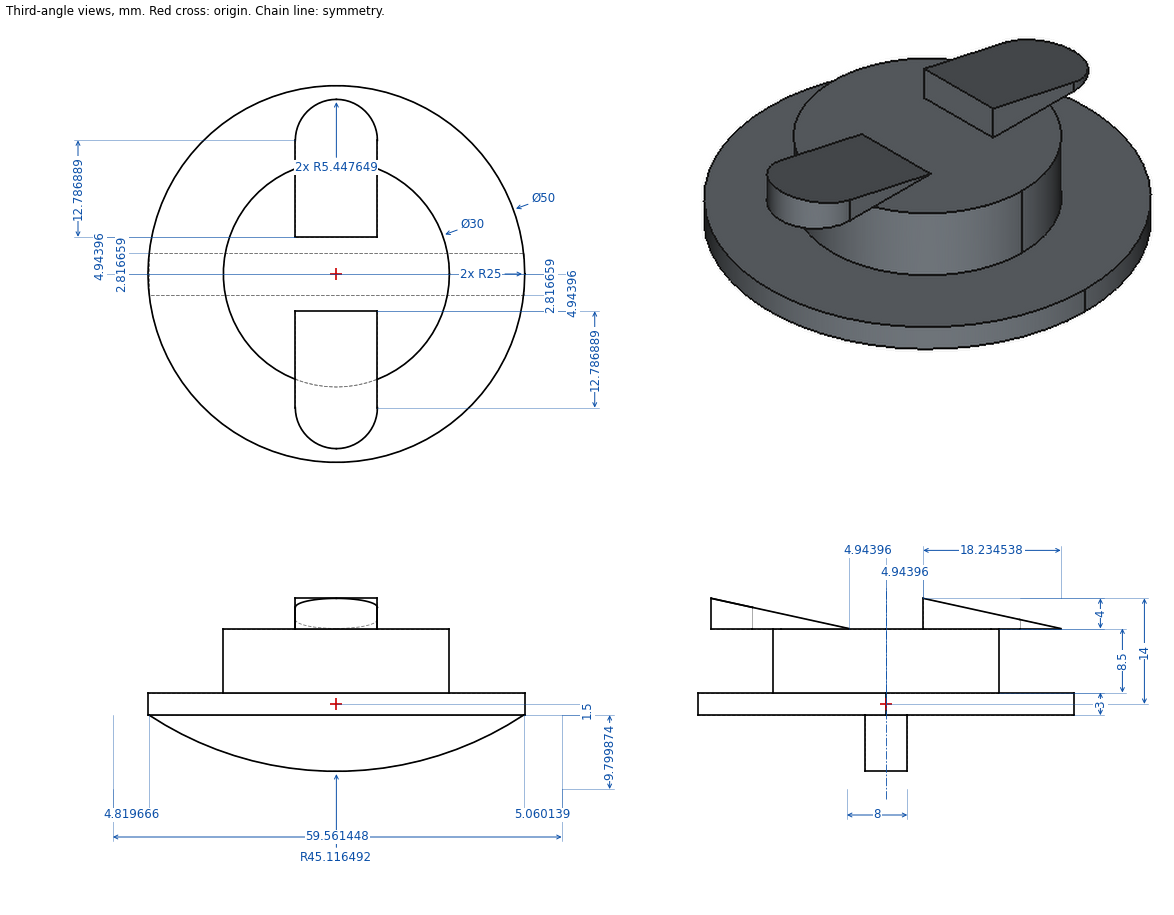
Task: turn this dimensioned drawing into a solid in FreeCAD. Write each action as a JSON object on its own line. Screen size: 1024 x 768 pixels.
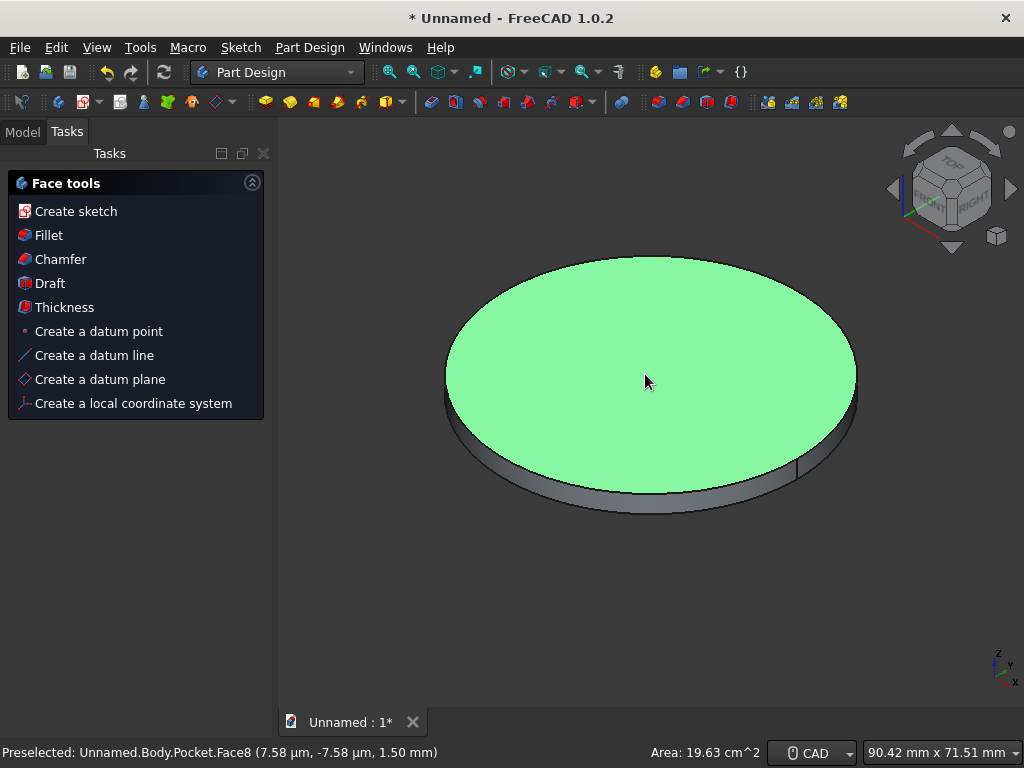
{"action": "left_click", "coordinate": [84, 102]}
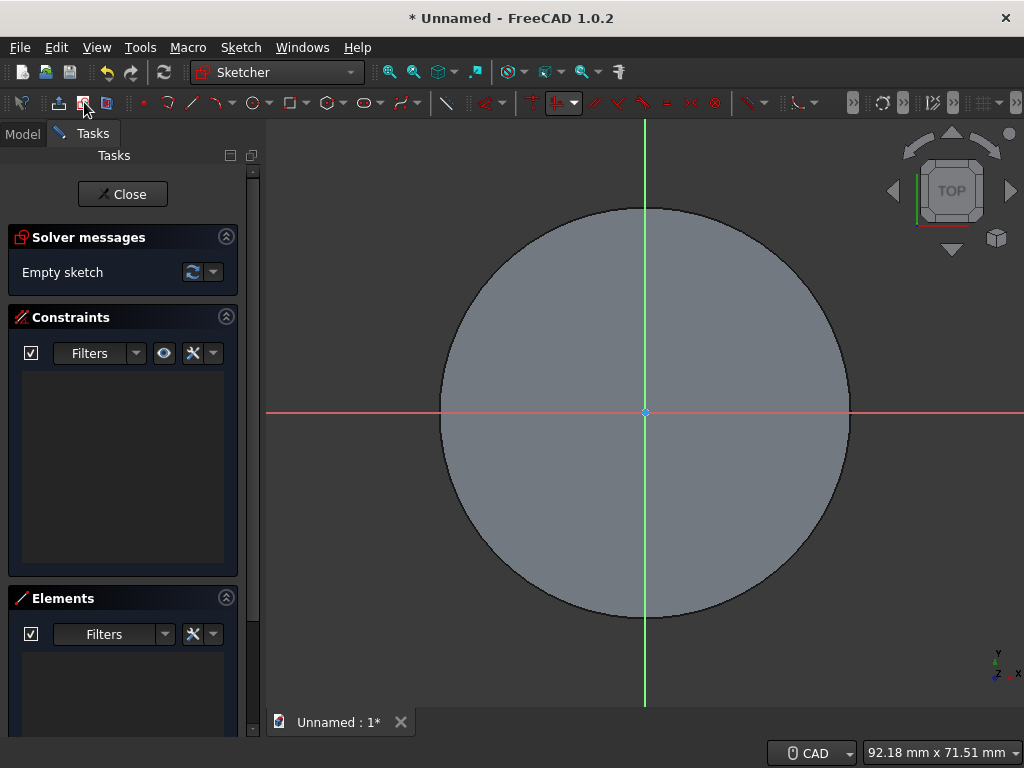
{"action": "scroll", "coordinate": [784, 413], "scroll_direction": "up", "scroll_amount": 2}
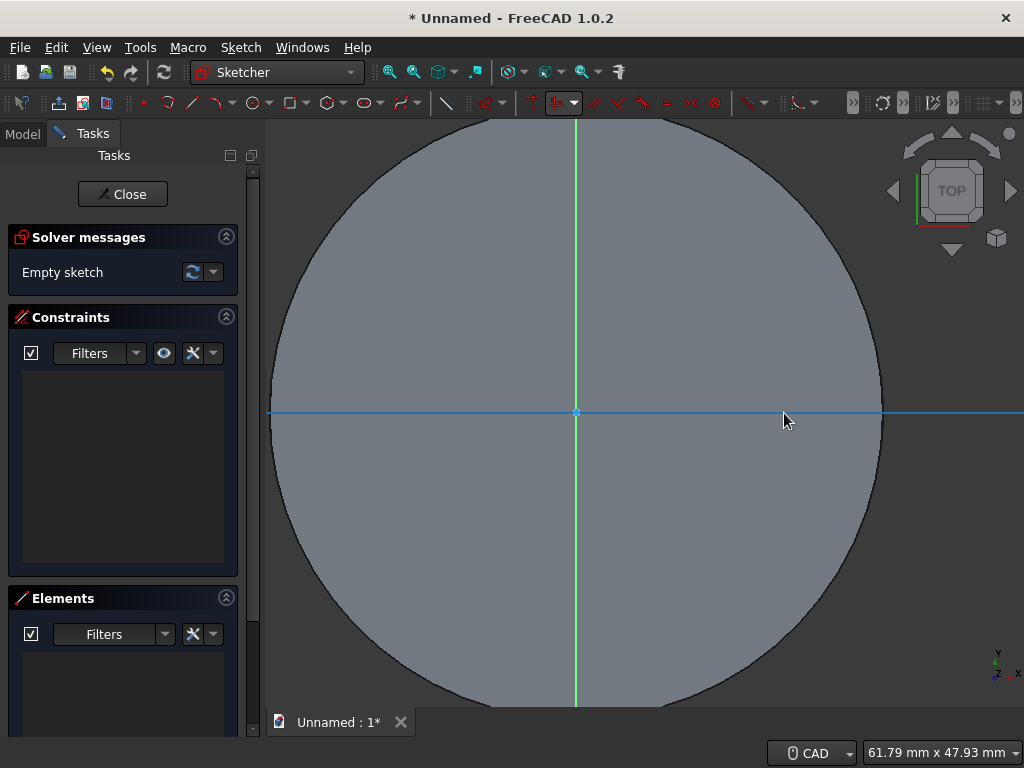
{"action": "key", "text": "g c"}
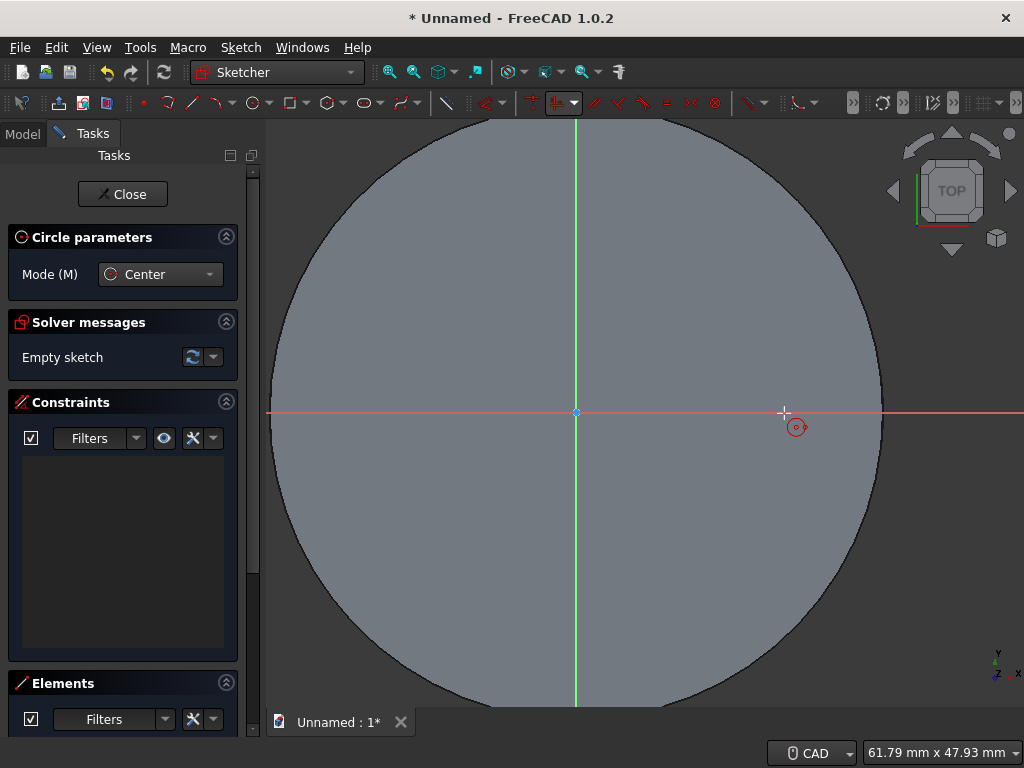
{"action": "left_click", "coordinate": [576, 413]}
{"action": "left_click", "coordinate": [706, 283]}
{"action": "key", "text": "Escape"}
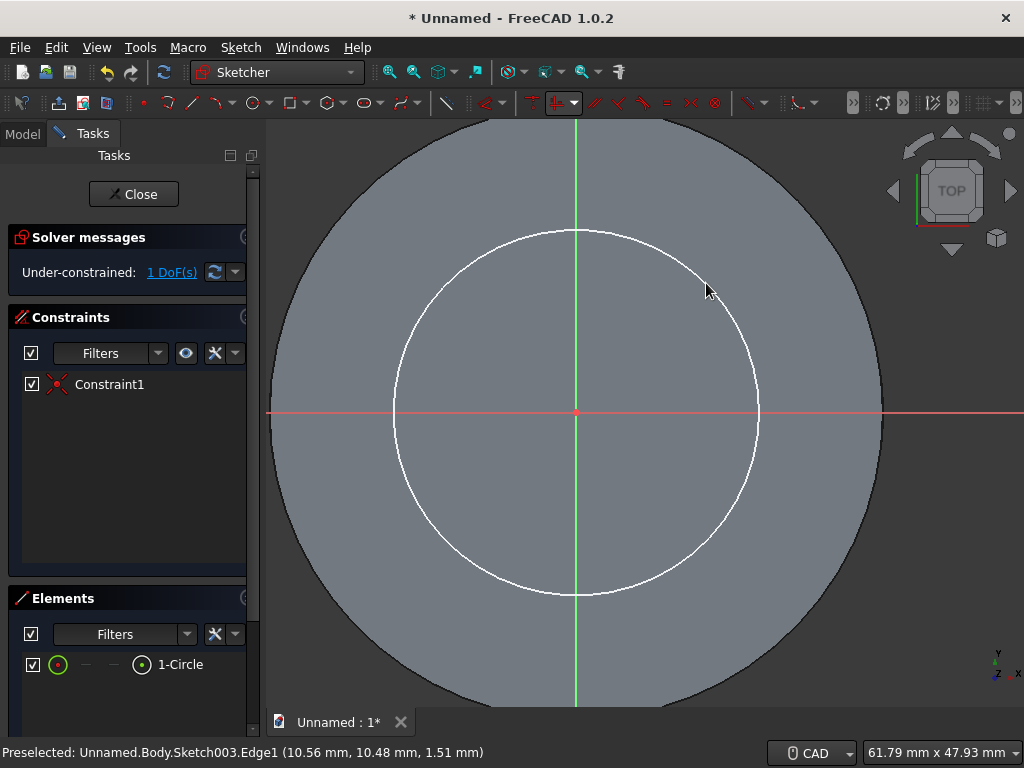
{"action": "left_click", "coordinate": [486, 104]}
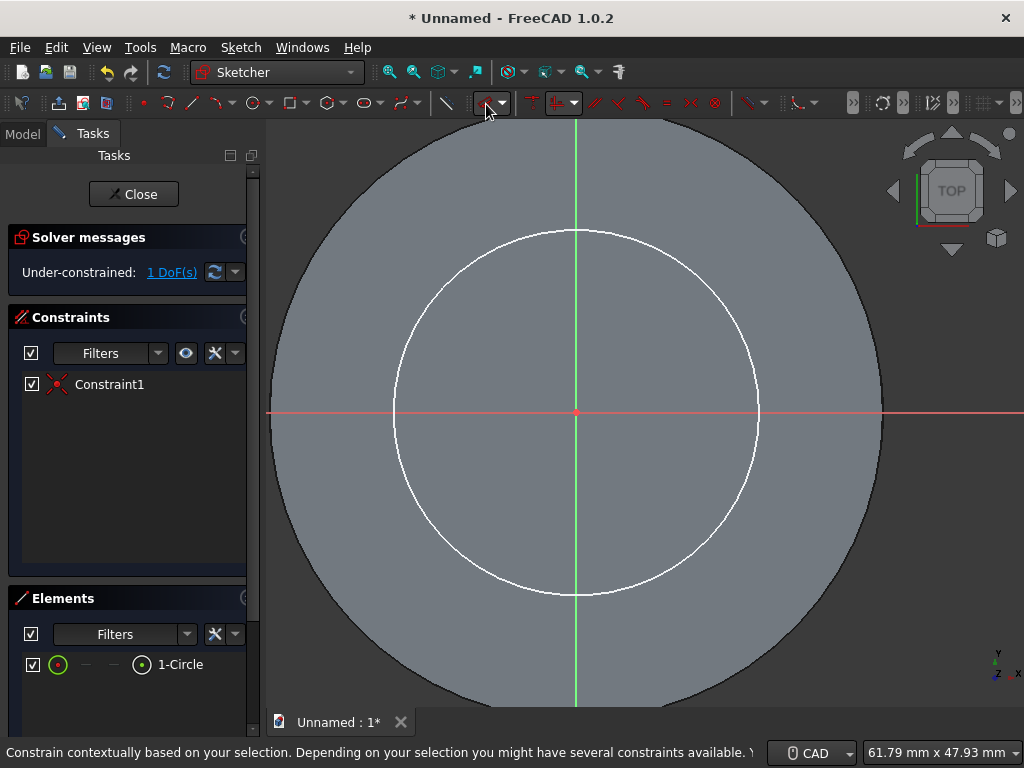
{"action": "left_click", "coordinate": [705, 283]}
{"action": "left_click", "coordinate": [728, 260]}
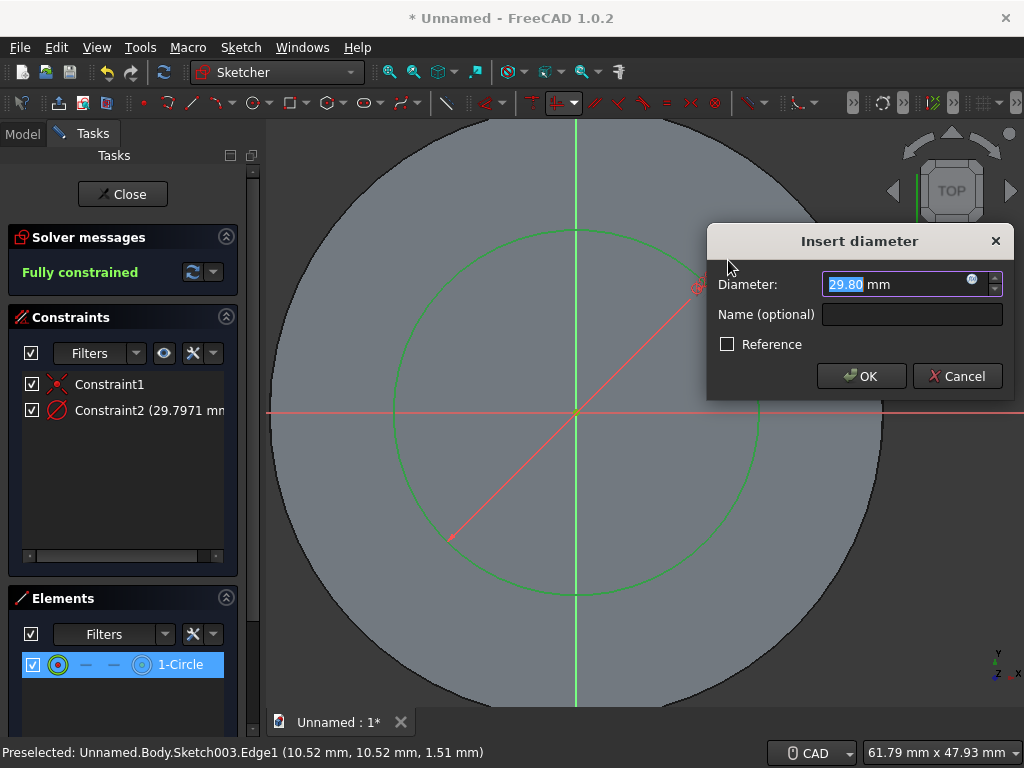
{"action": "type", "text": "30"}
{"action": "key", "text": "Return"}
{"action": "key", "text": "Escape"}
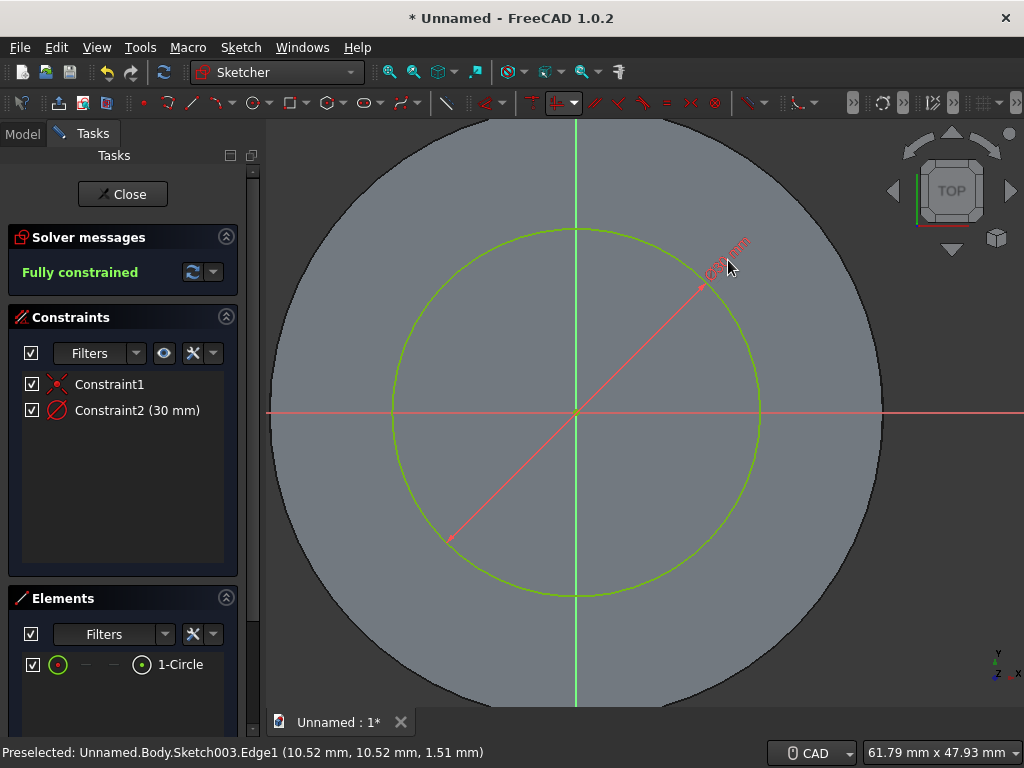
{"action": "left_click", "coordinate": [123, 194]}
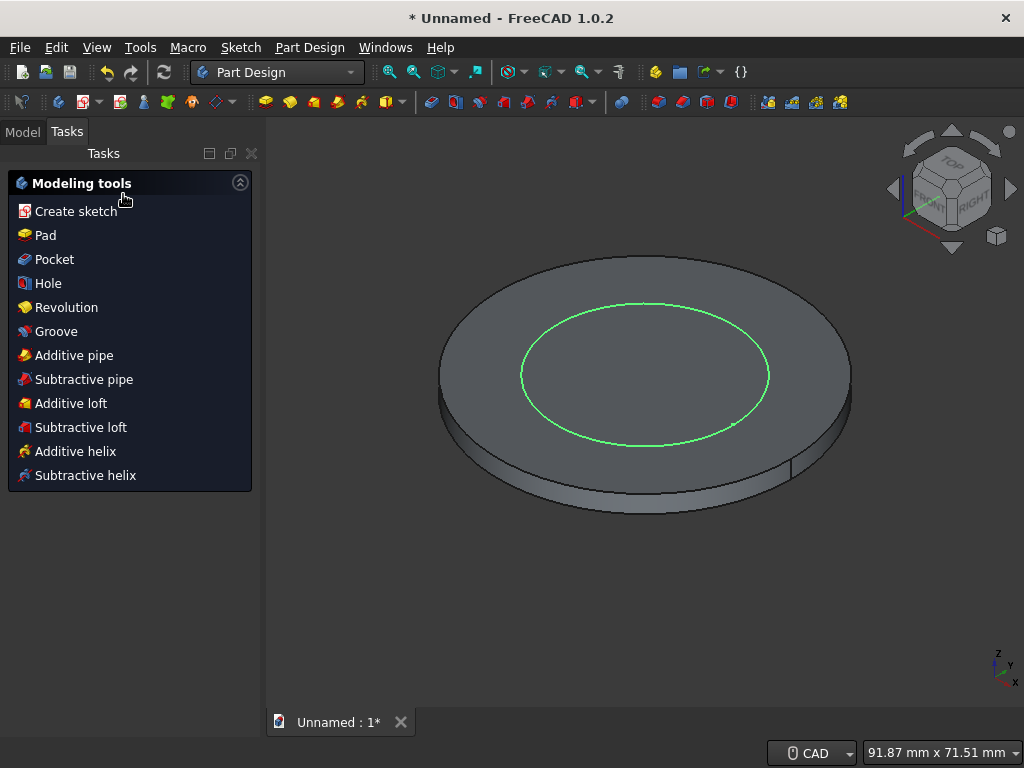
{"action": "left_click", "coordinate": [266, 102]}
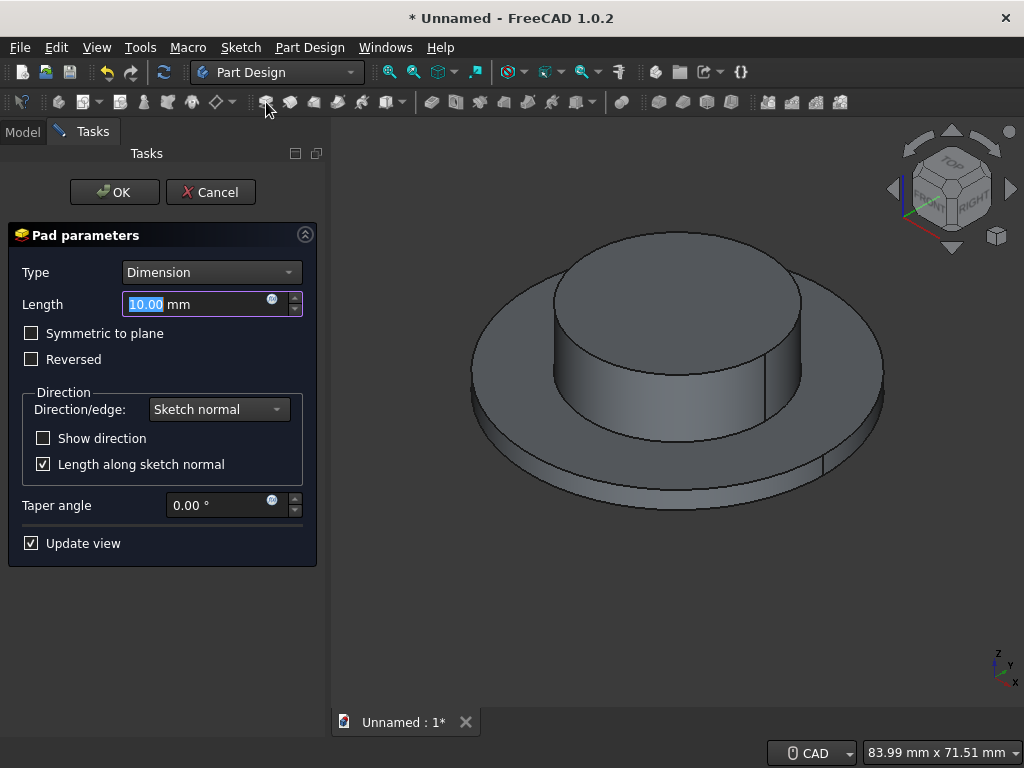
{"action": "type", "text": "8.5"}
{"action": "key", "text": "Tab"}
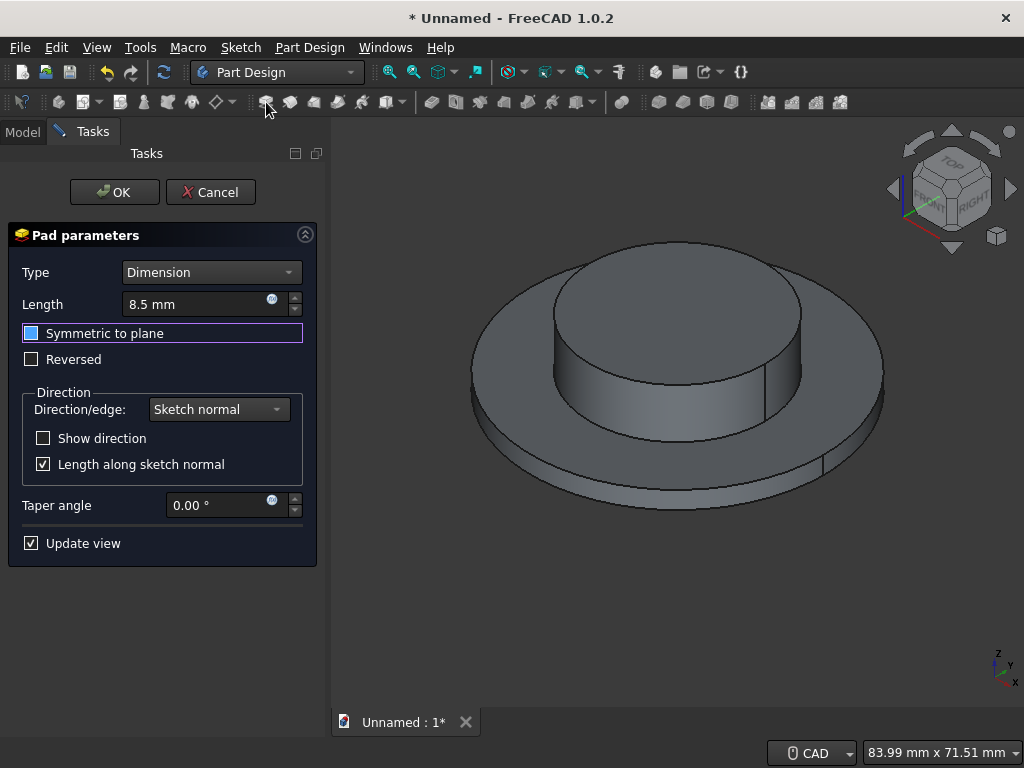
{"action": "left_click", "coordinate": [115, 192]}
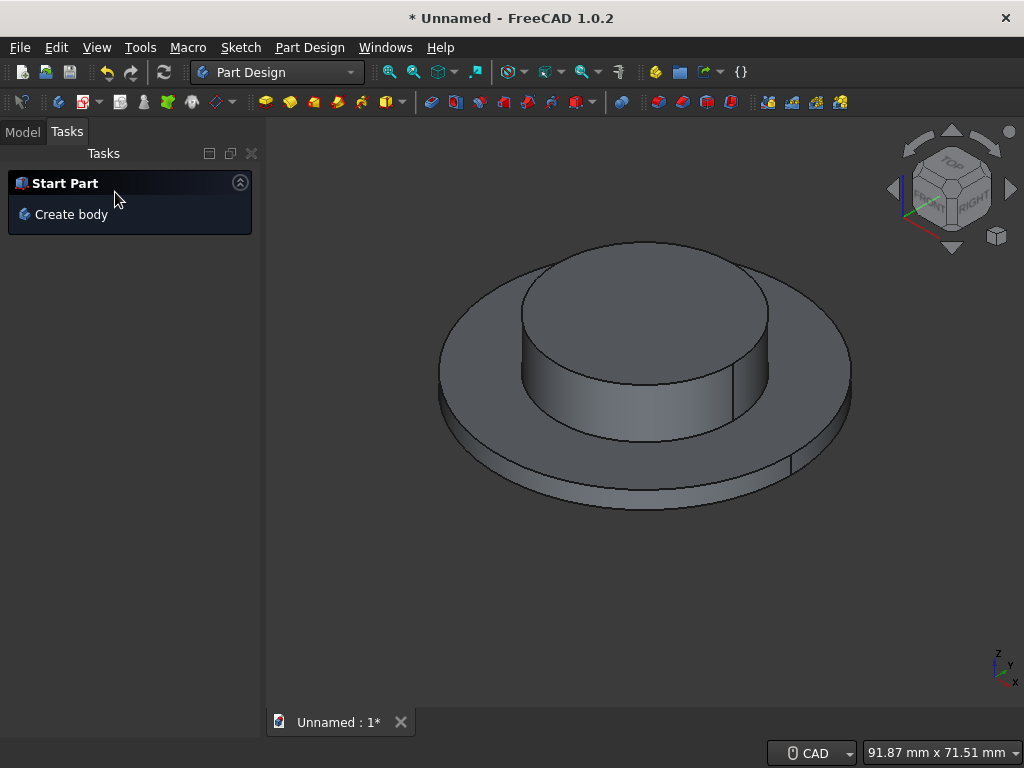
{"action": "left_click", "coordinate": [645, 313]}